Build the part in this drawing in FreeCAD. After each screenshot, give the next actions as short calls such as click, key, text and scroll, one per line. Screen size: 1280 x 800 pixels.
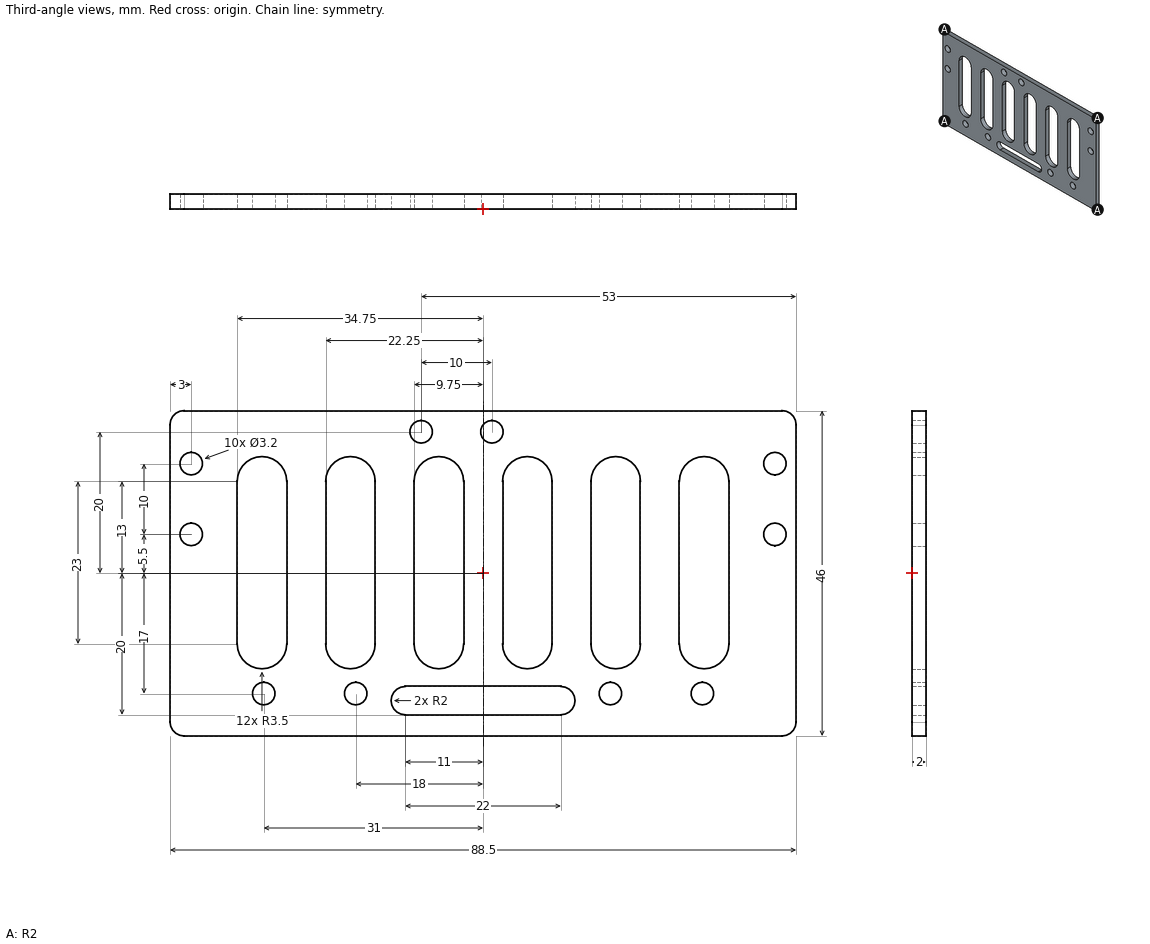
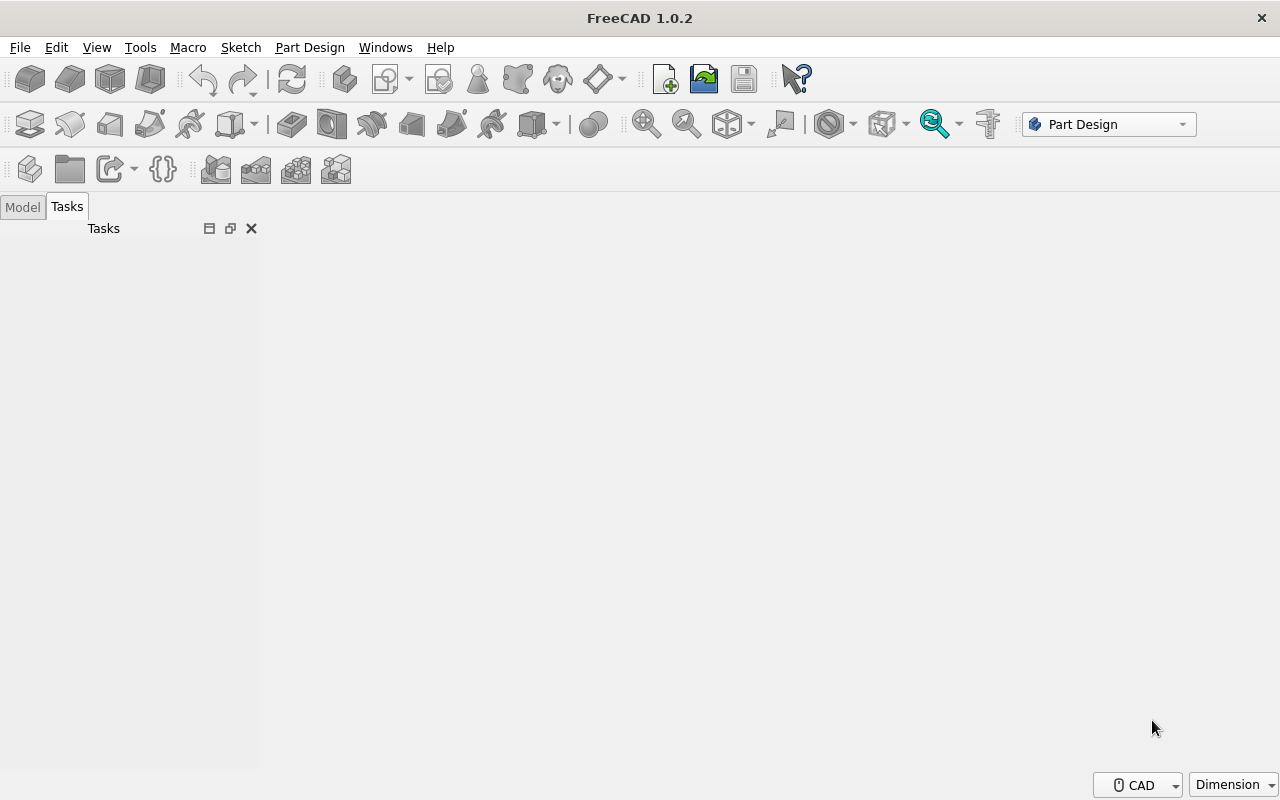
click(664, 80)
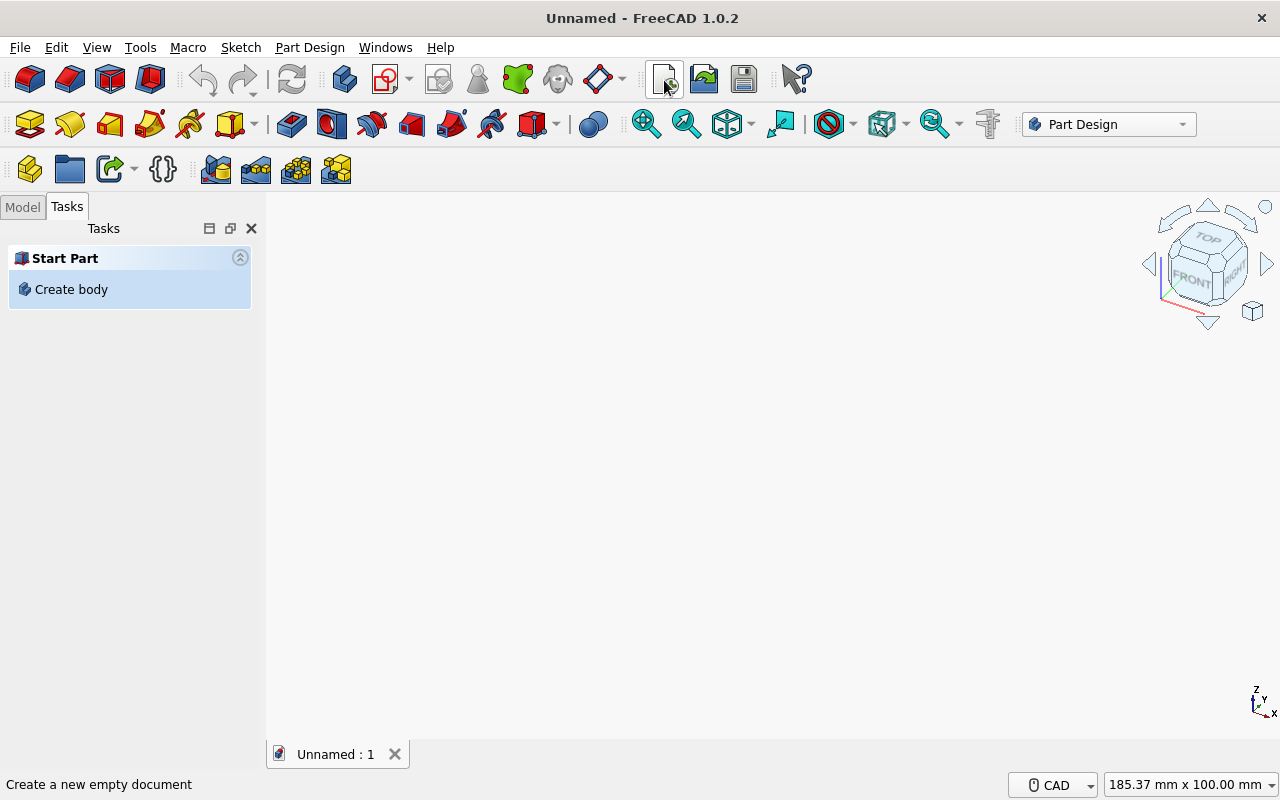
click(386, 80)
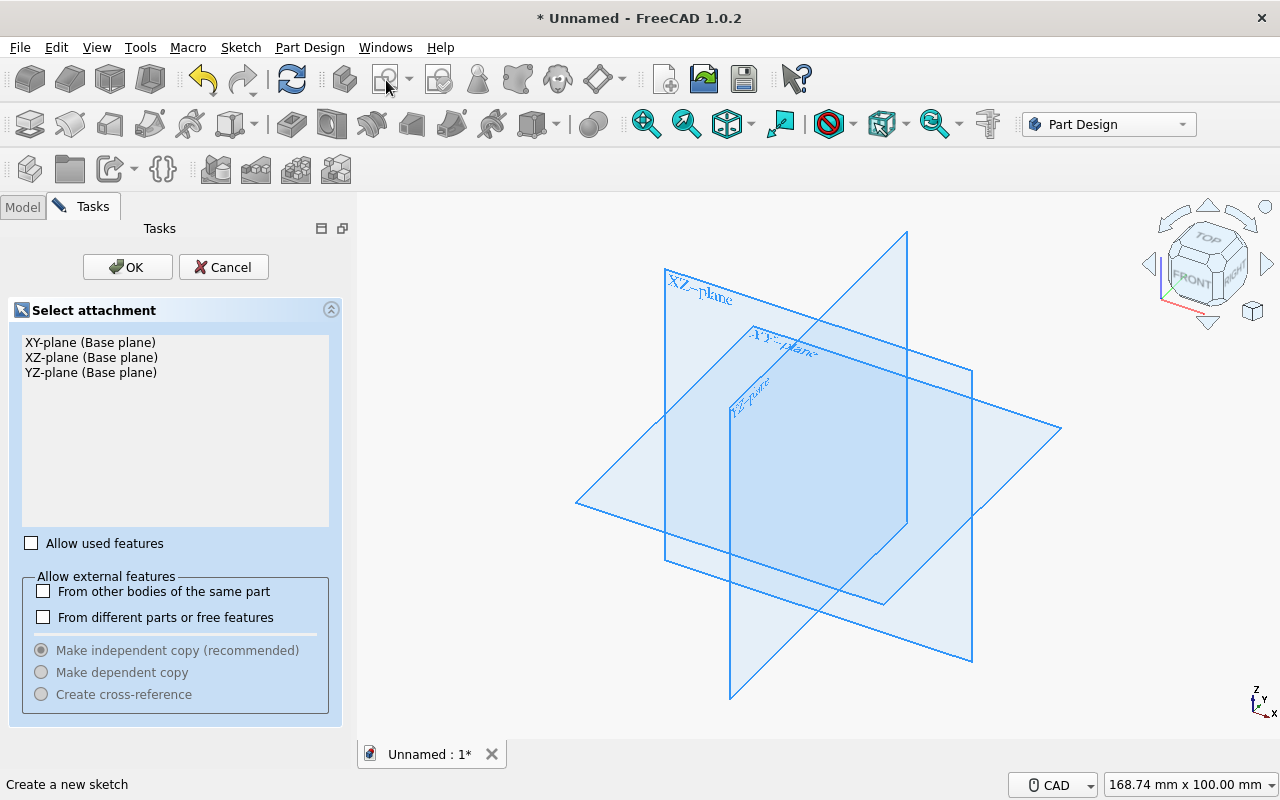
click(82, 358)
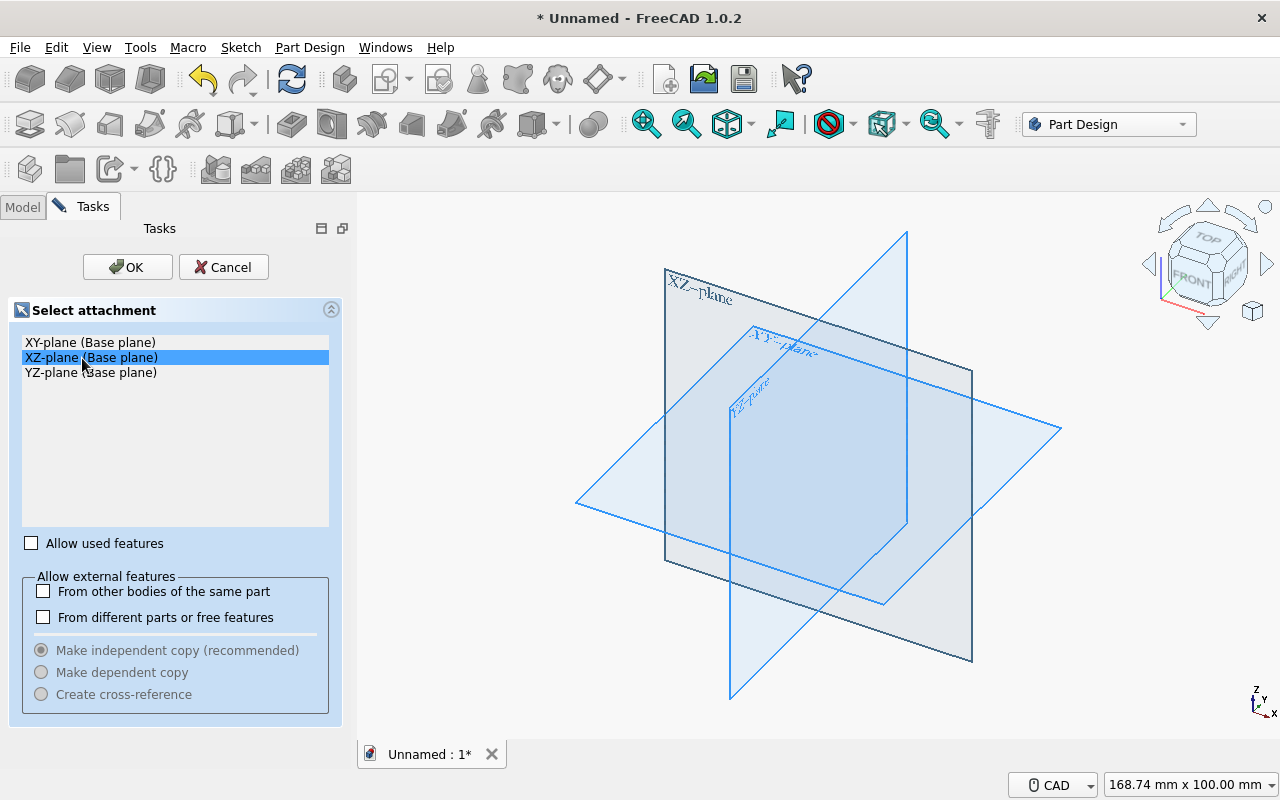
click(128, 267)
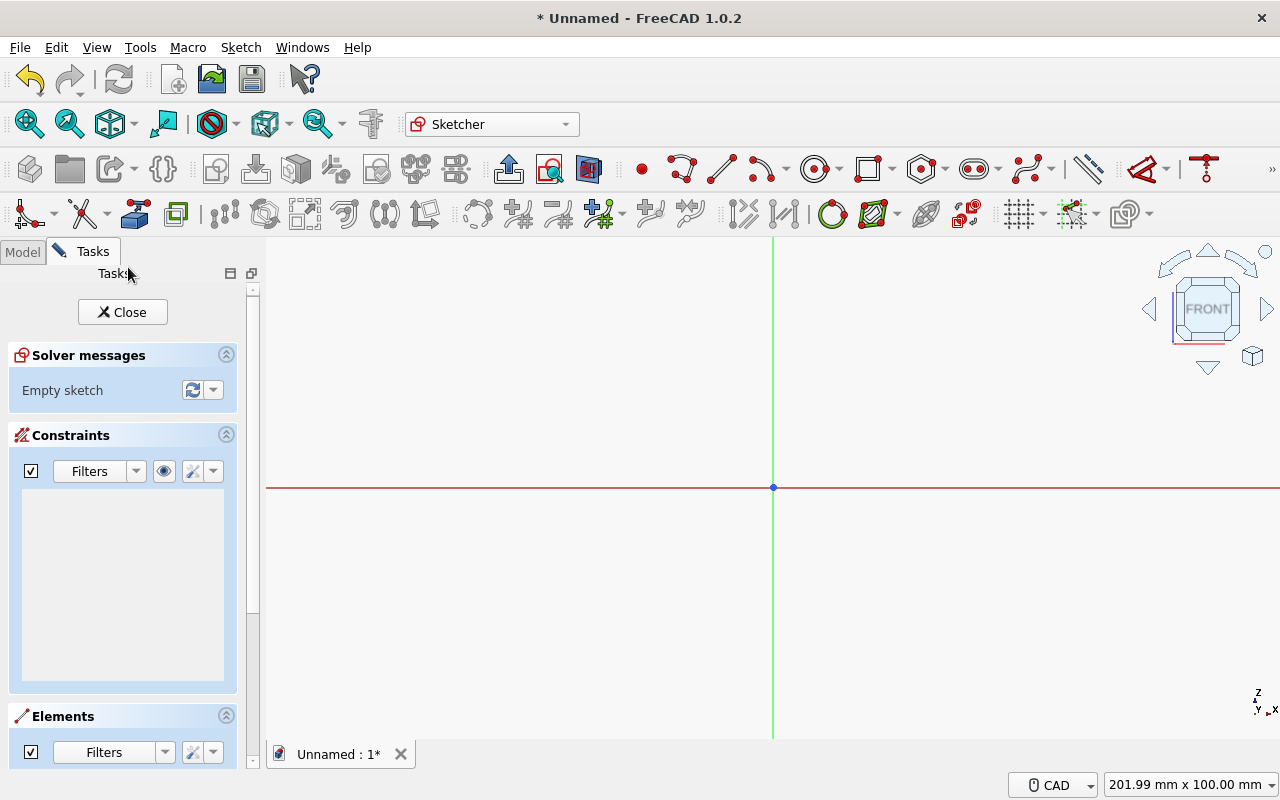
key(g)
key(v)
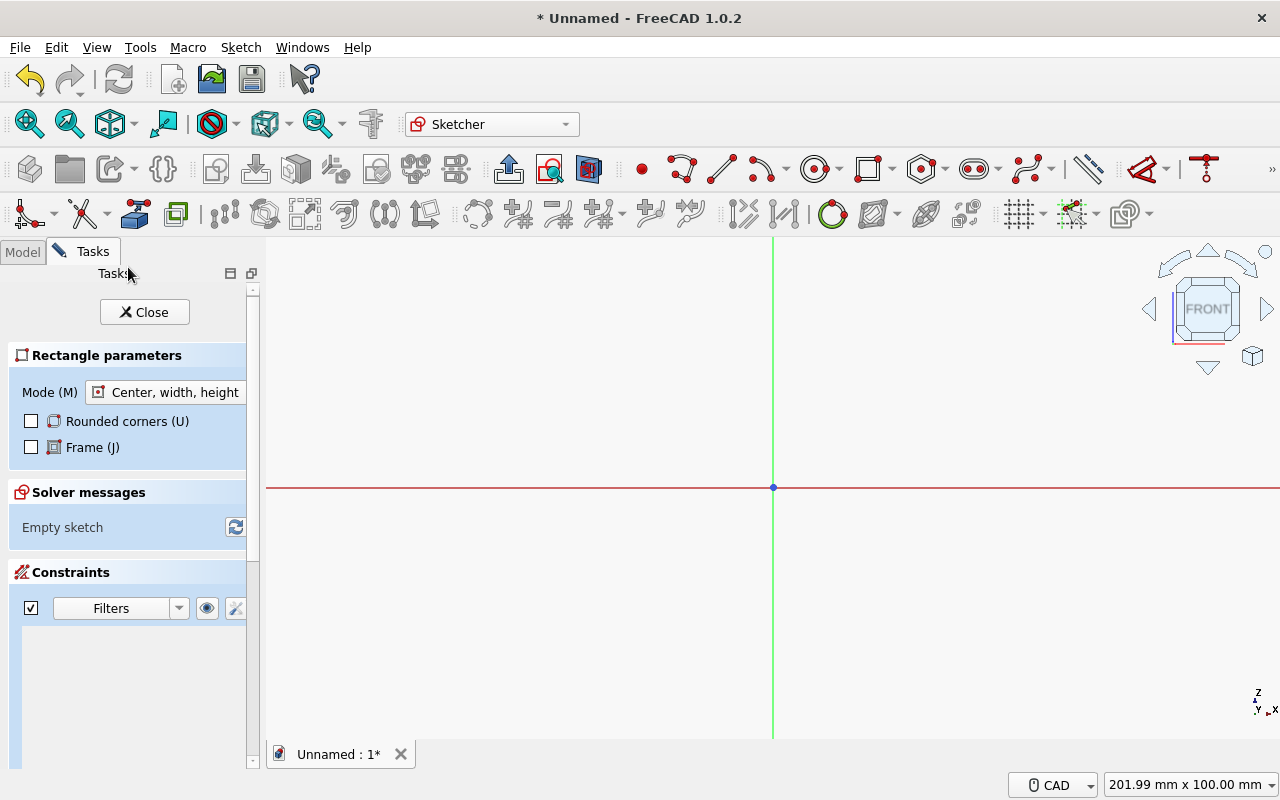
click(773, 488)
move(995, 373)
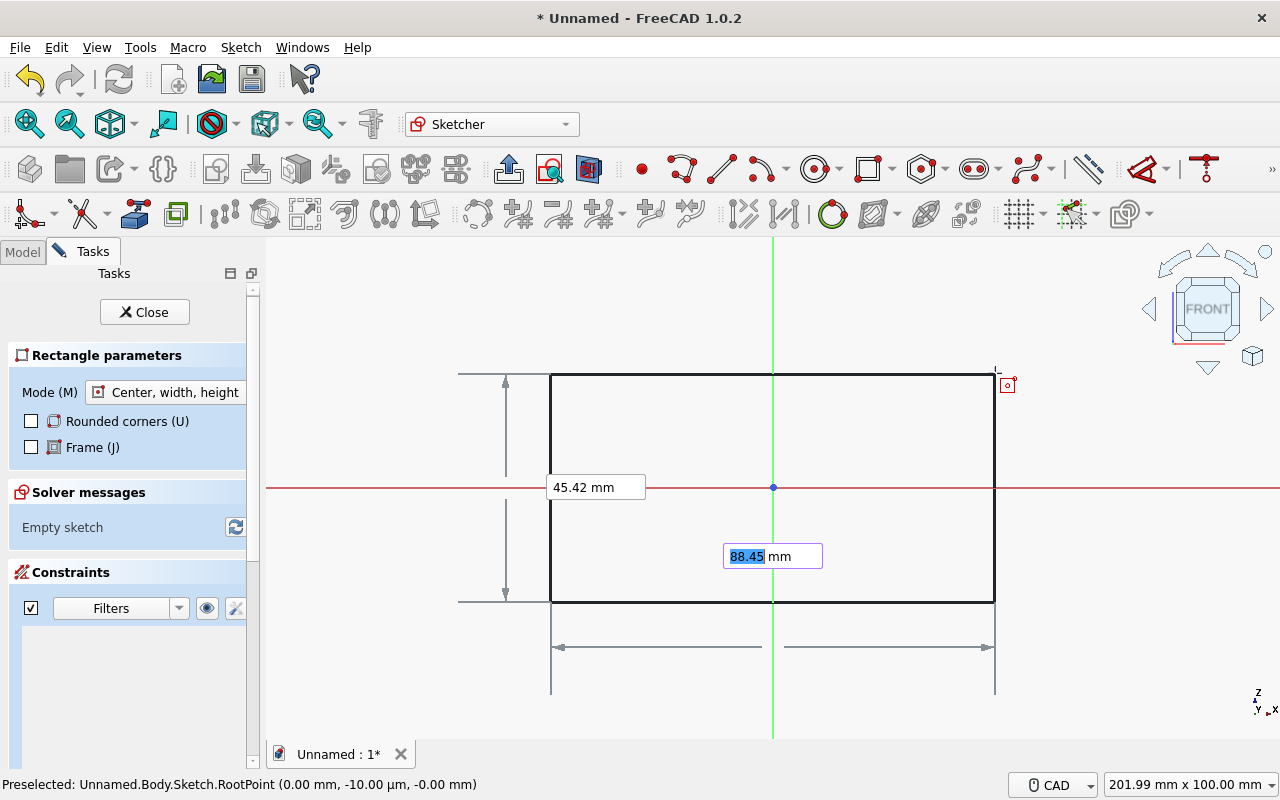
text(88.5)
key(Tab)
text(46)
key(Return)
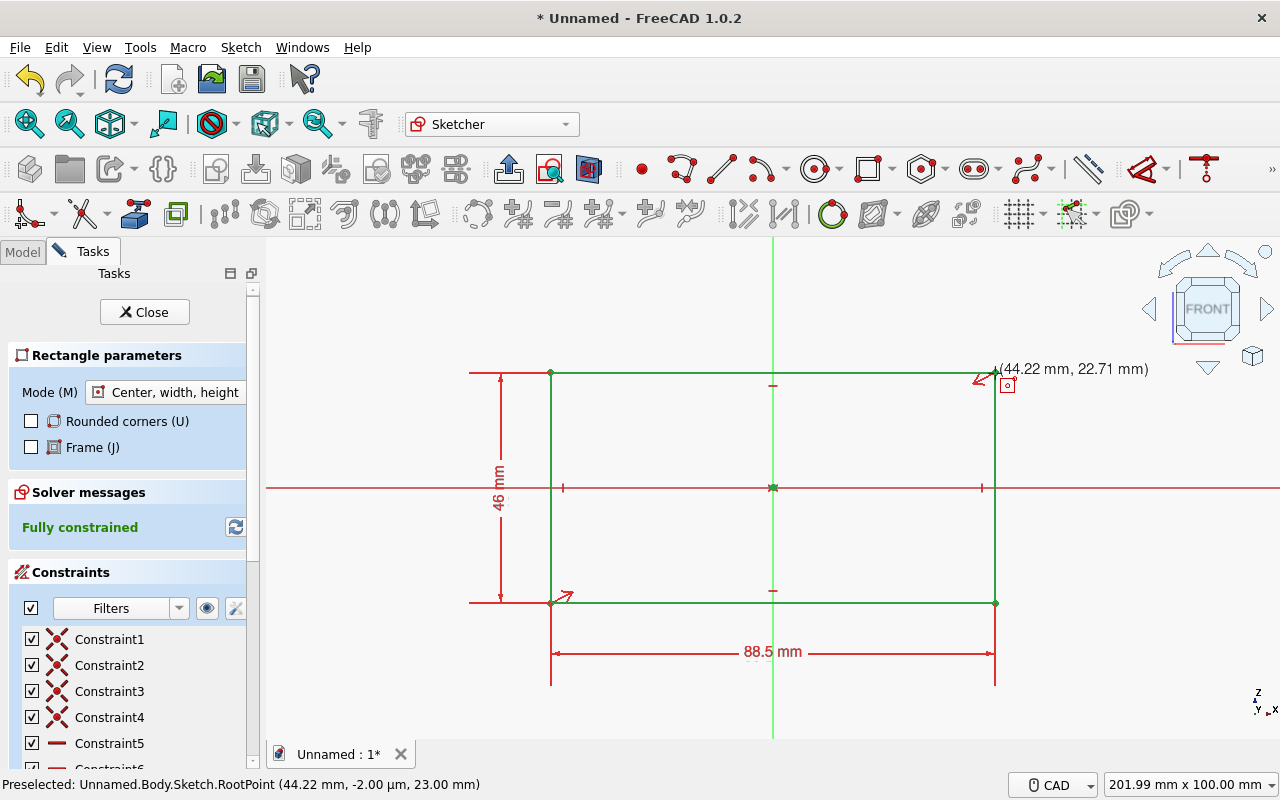
click(816, 170)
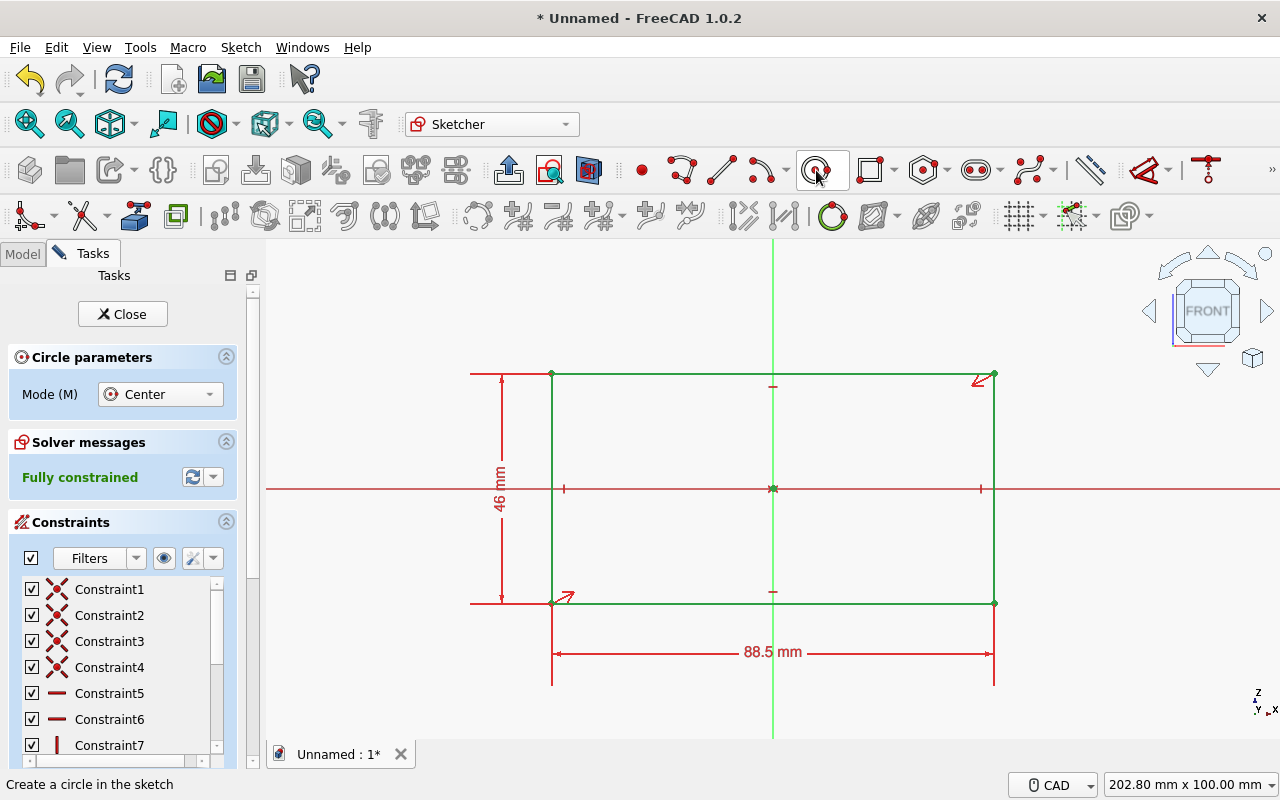
scroll(567, 412, up, 6)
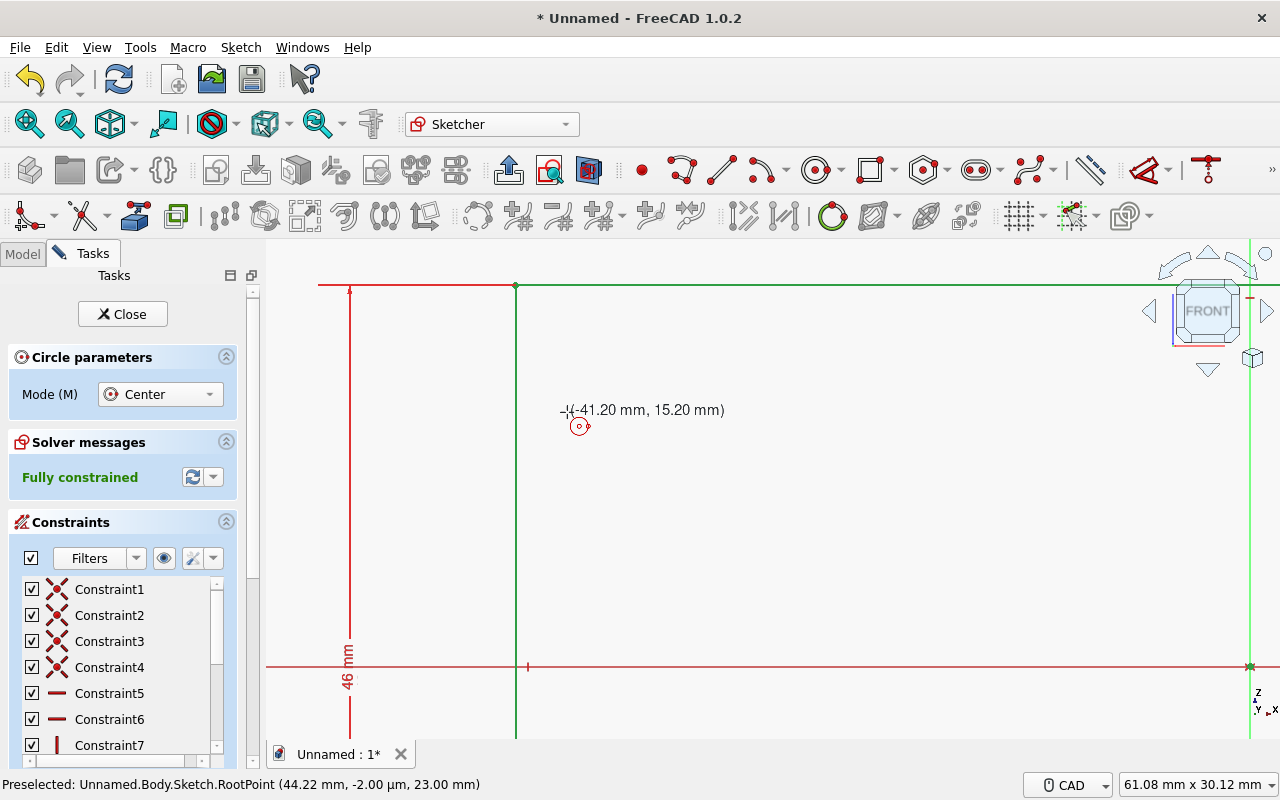
click(565, 410)
move(584, 391)